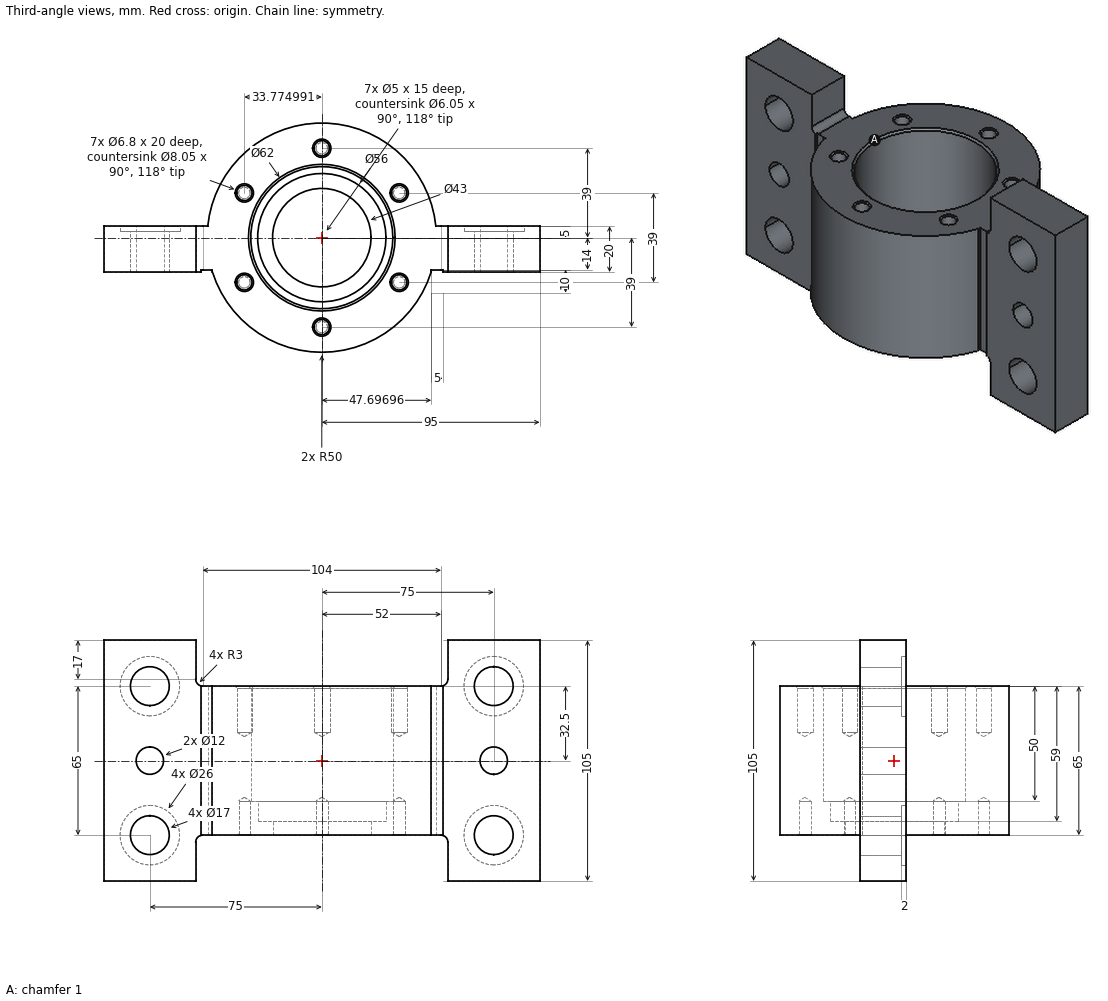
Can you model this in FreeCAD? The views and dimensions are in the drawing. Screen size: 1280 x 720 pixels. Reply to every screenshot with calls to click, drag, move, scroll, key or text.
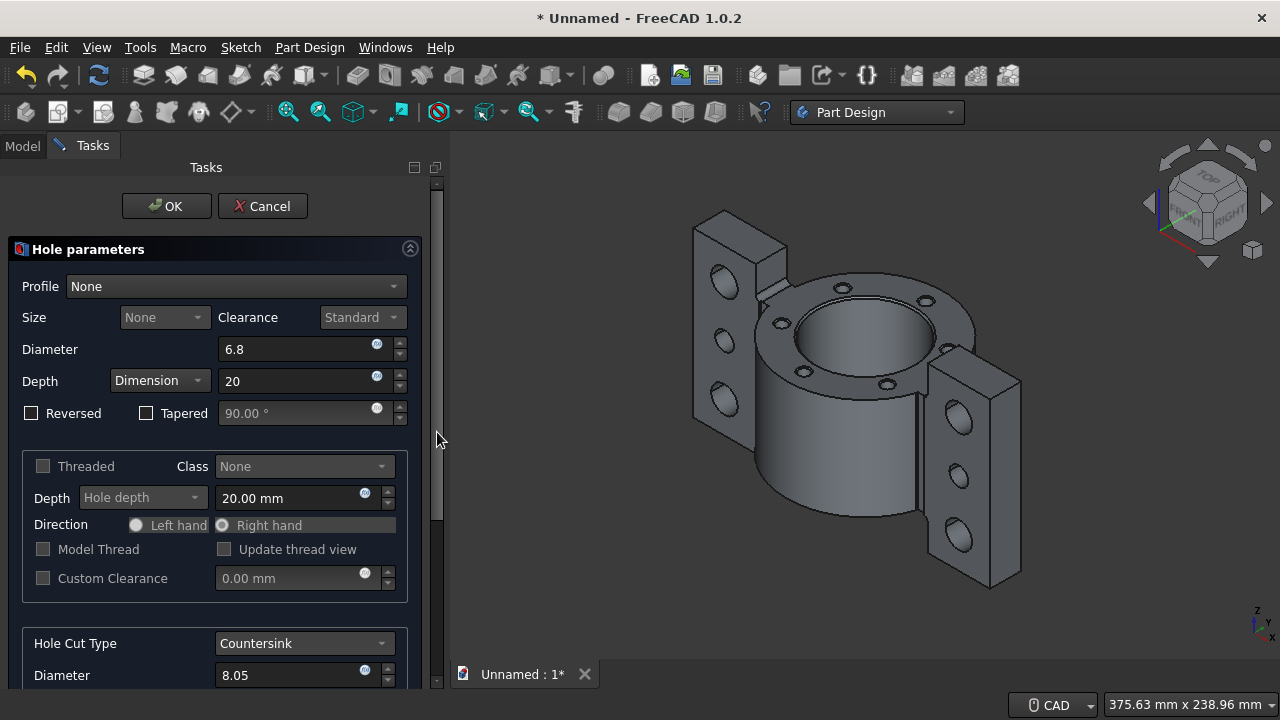
click(167, 206)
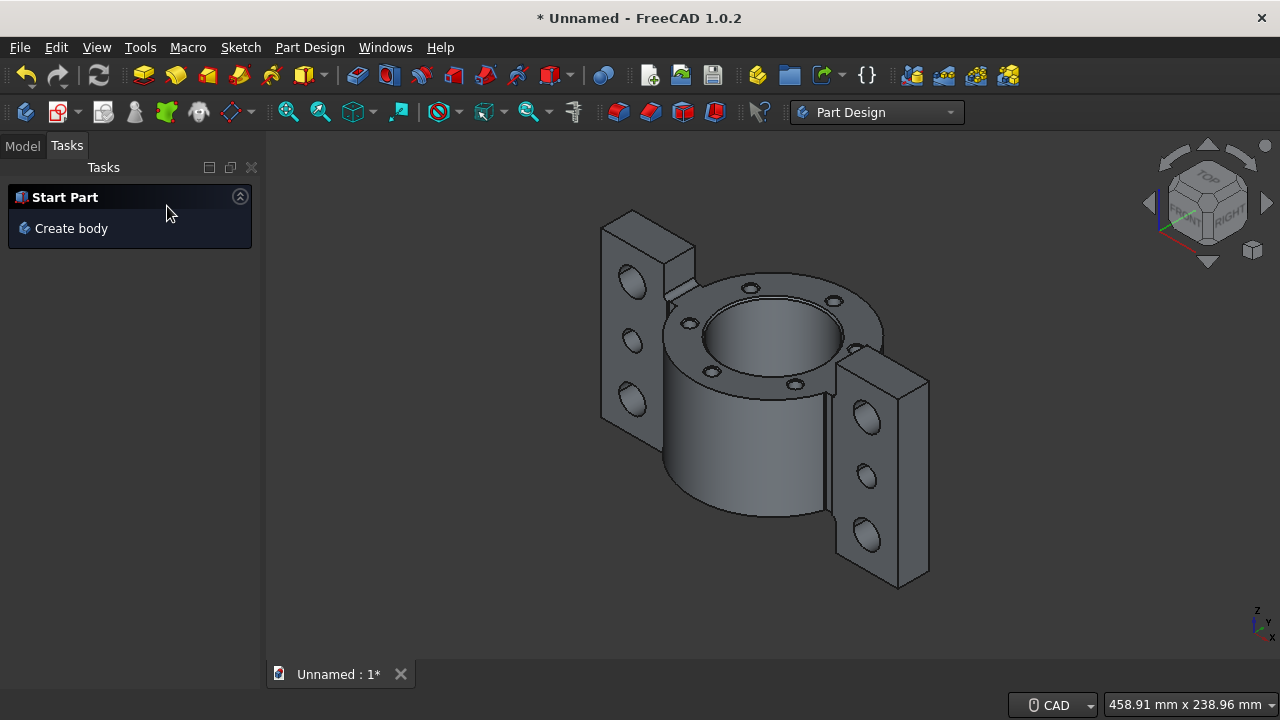
key(5)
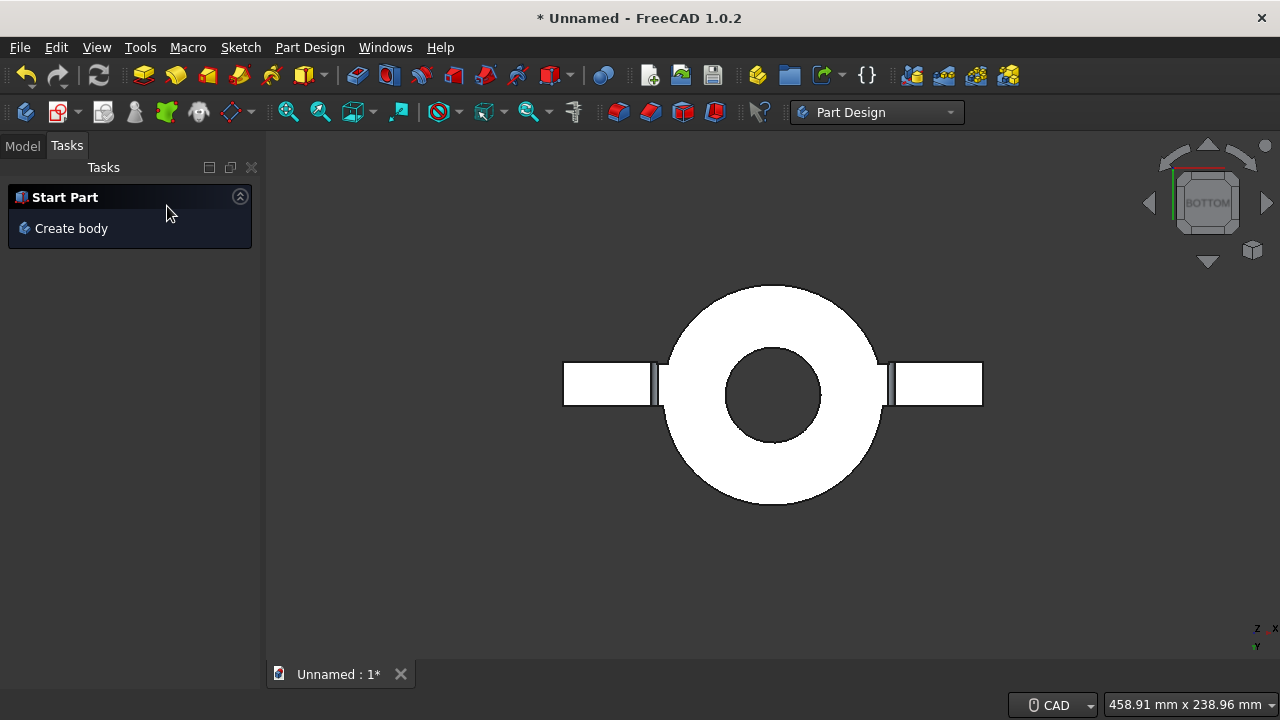
click(290, 112)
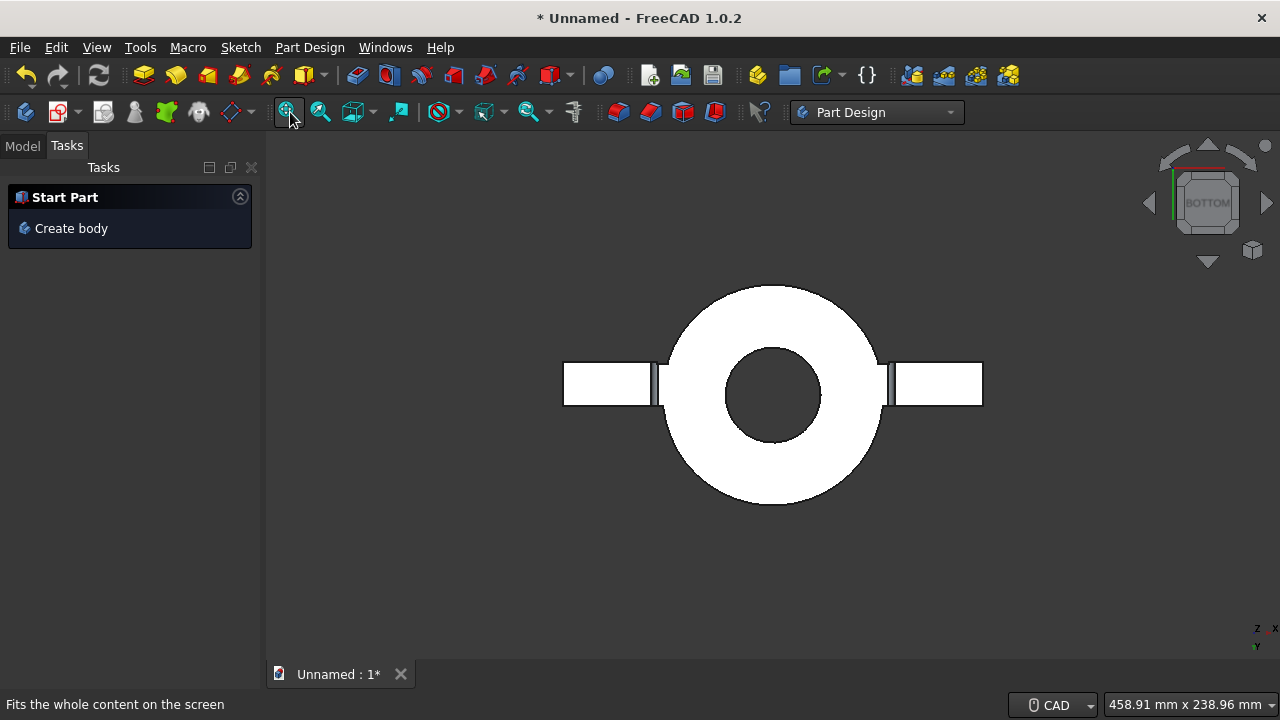
click(707, 363)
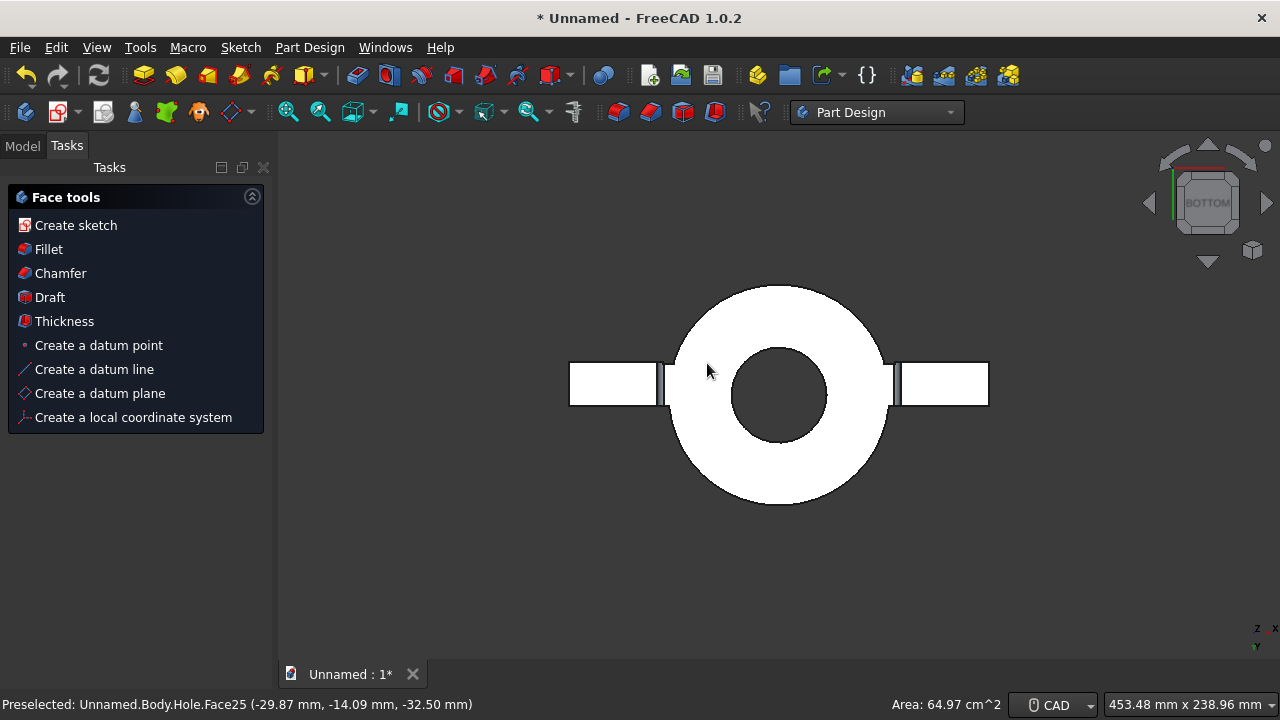
click(58, 112)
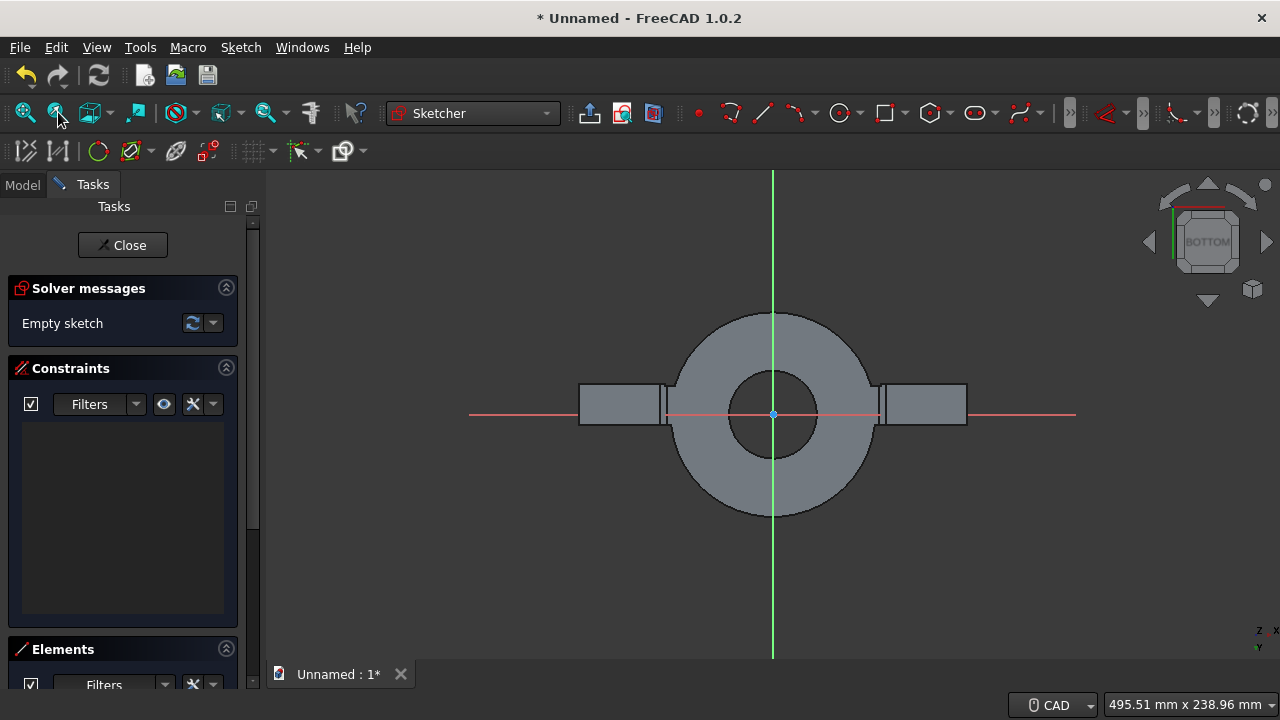
click(654, 114)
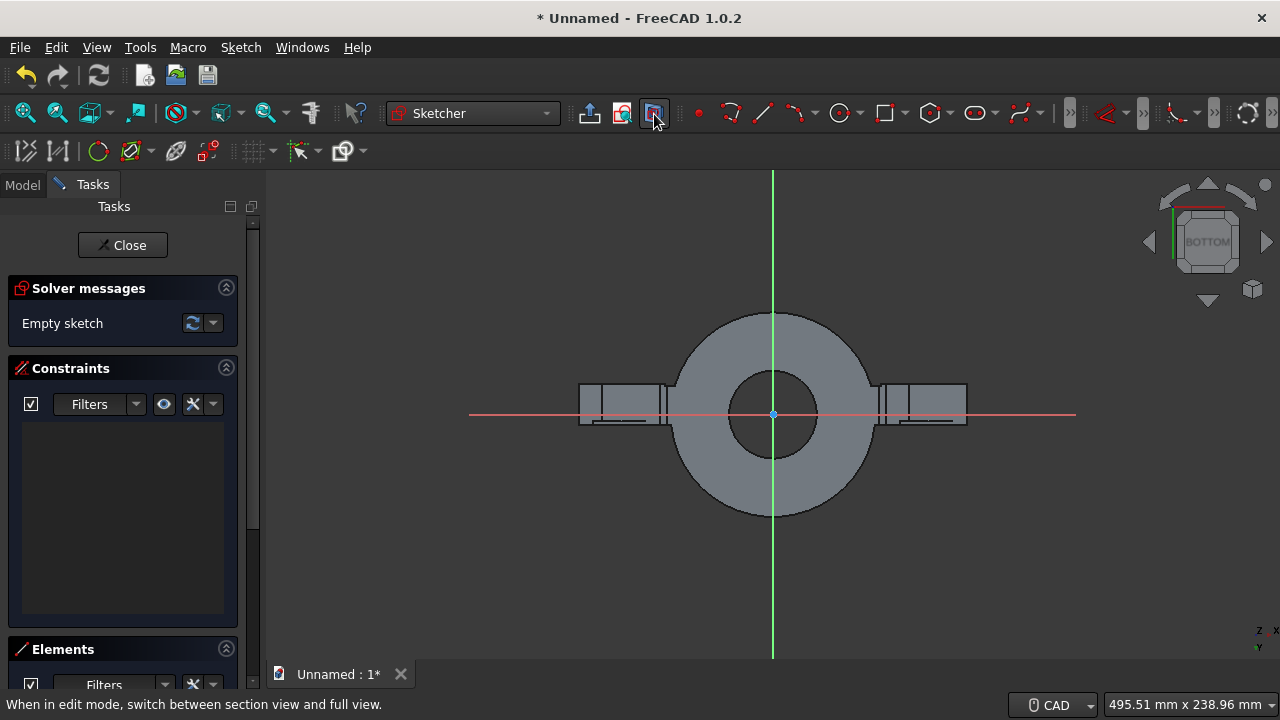
scroll(856, 415, up, 3)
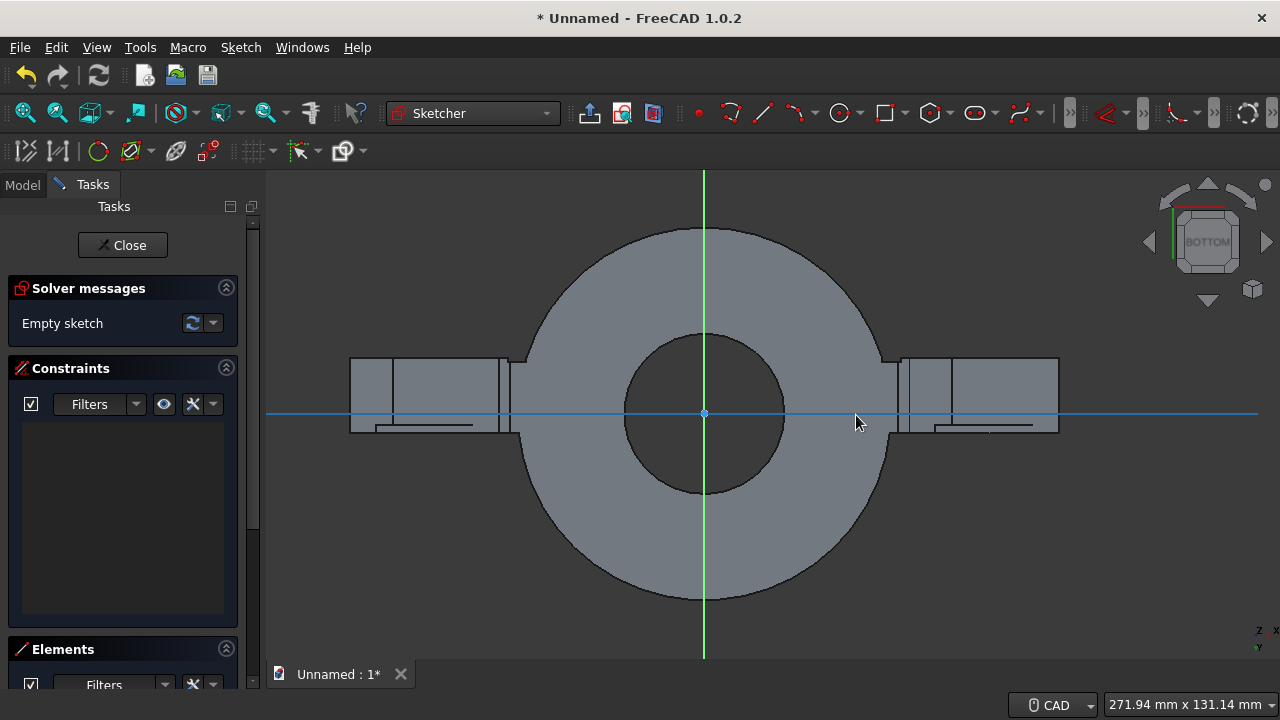
click(840, 114)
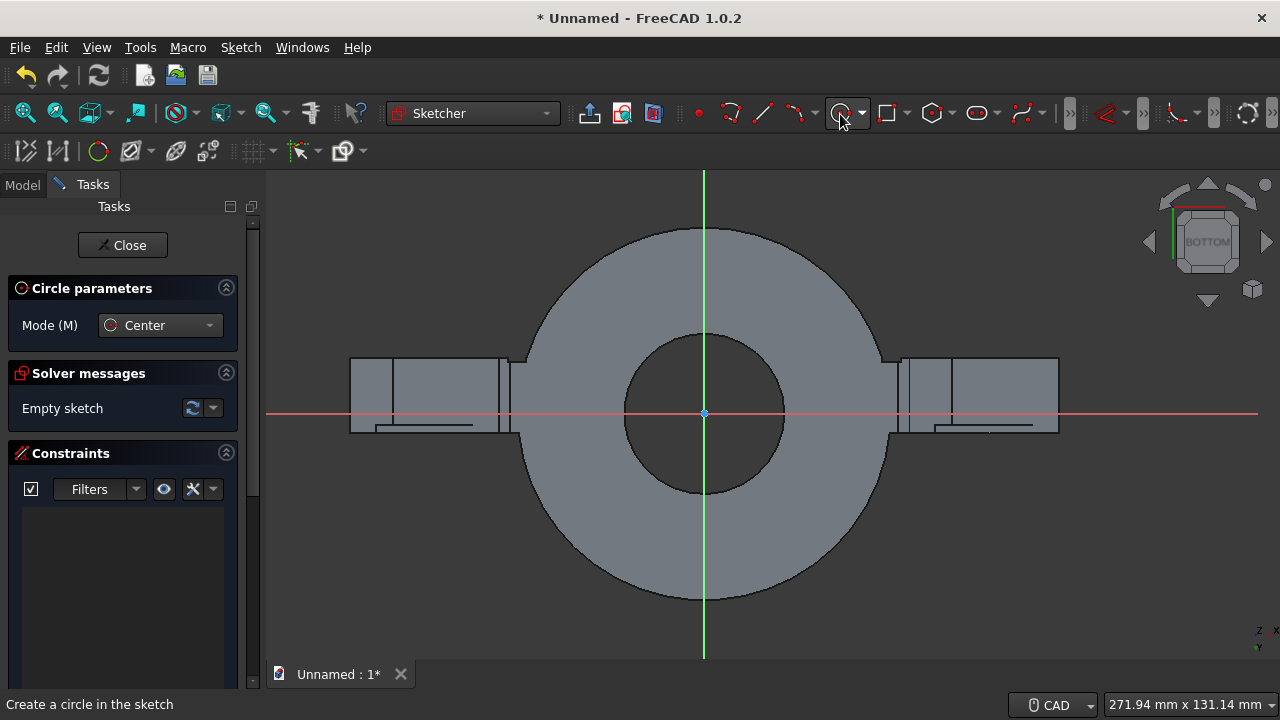
scroll(704, 414, up, 5)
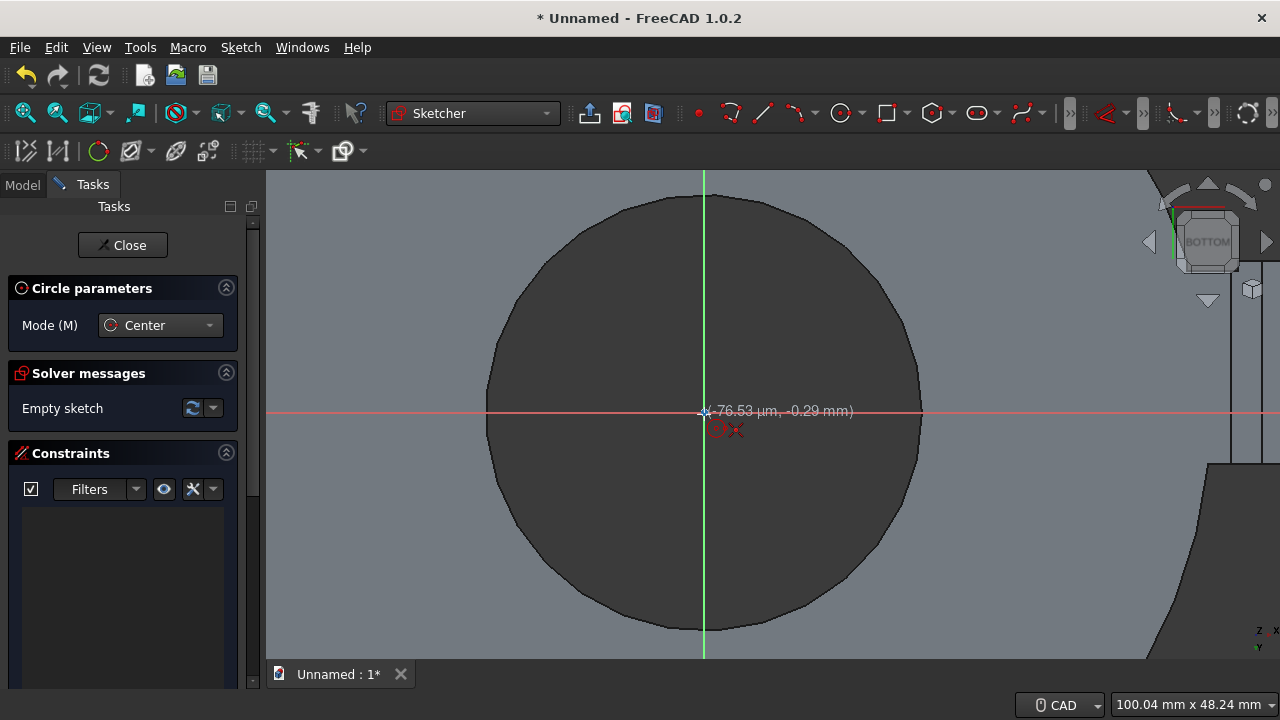
click(704, 413)
click(722, 395)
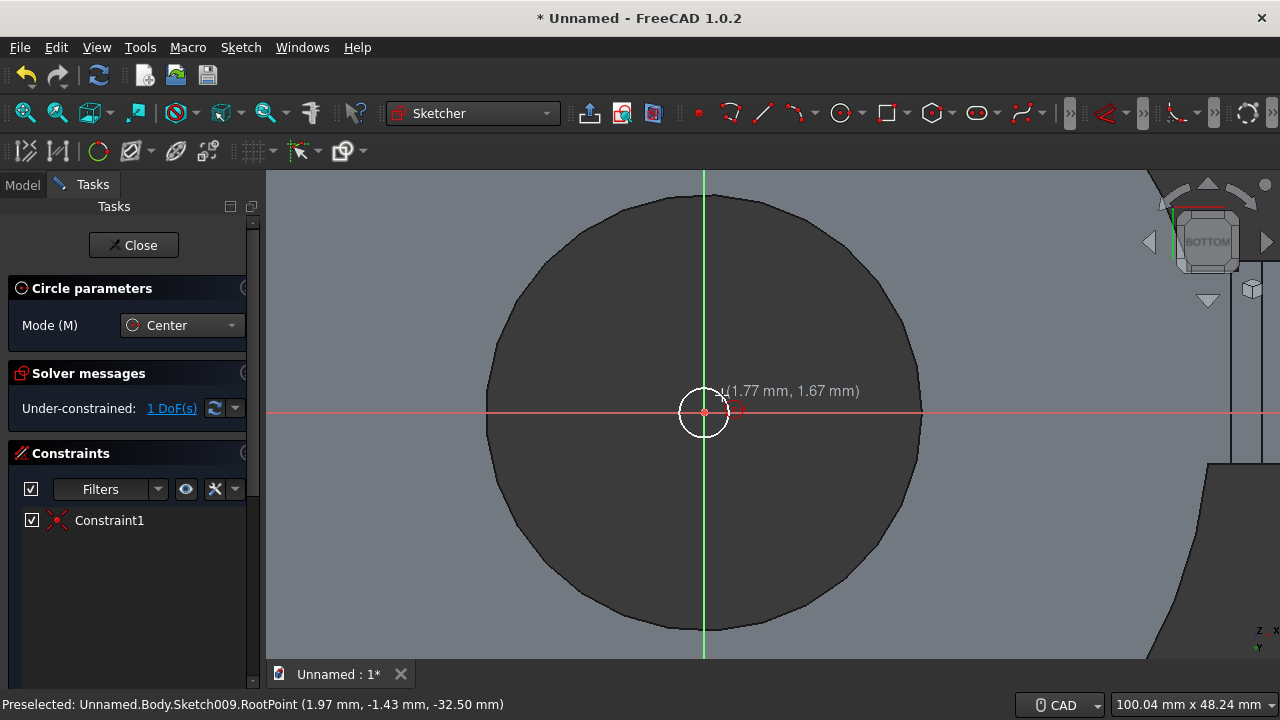
scroll(705, 415, down, 5)